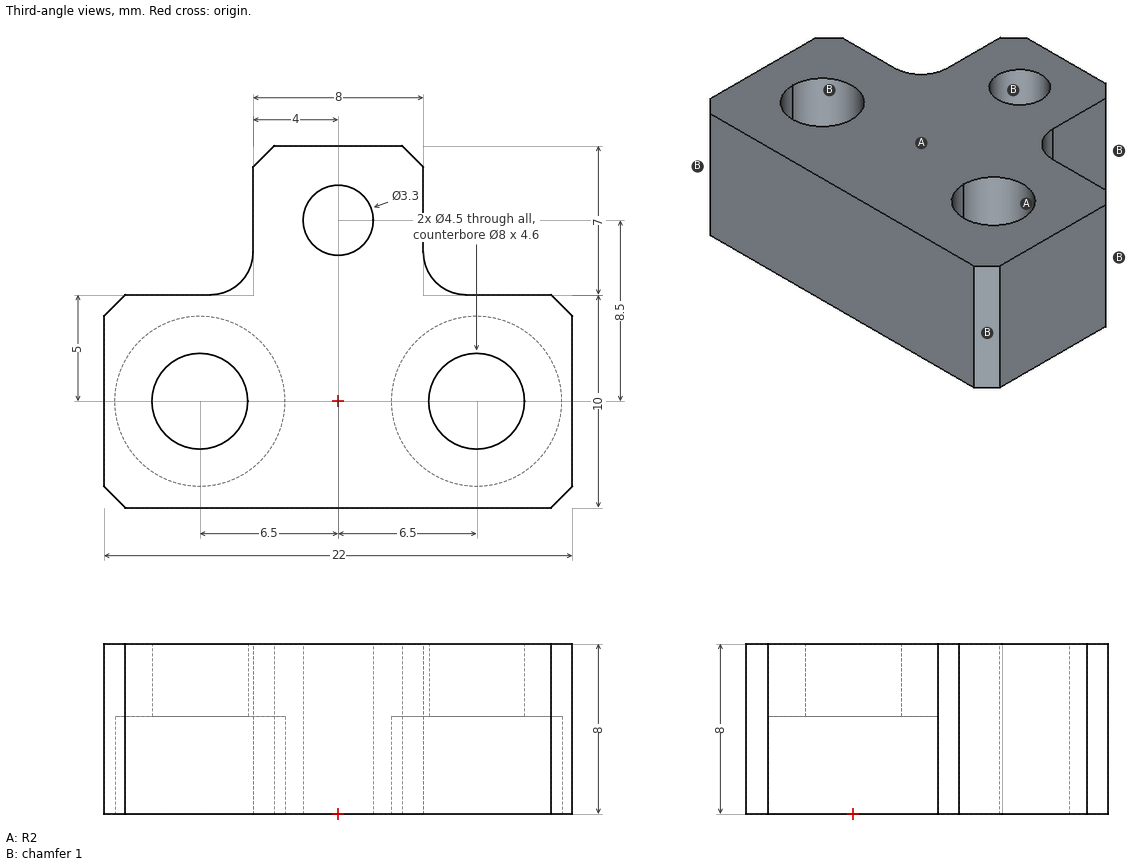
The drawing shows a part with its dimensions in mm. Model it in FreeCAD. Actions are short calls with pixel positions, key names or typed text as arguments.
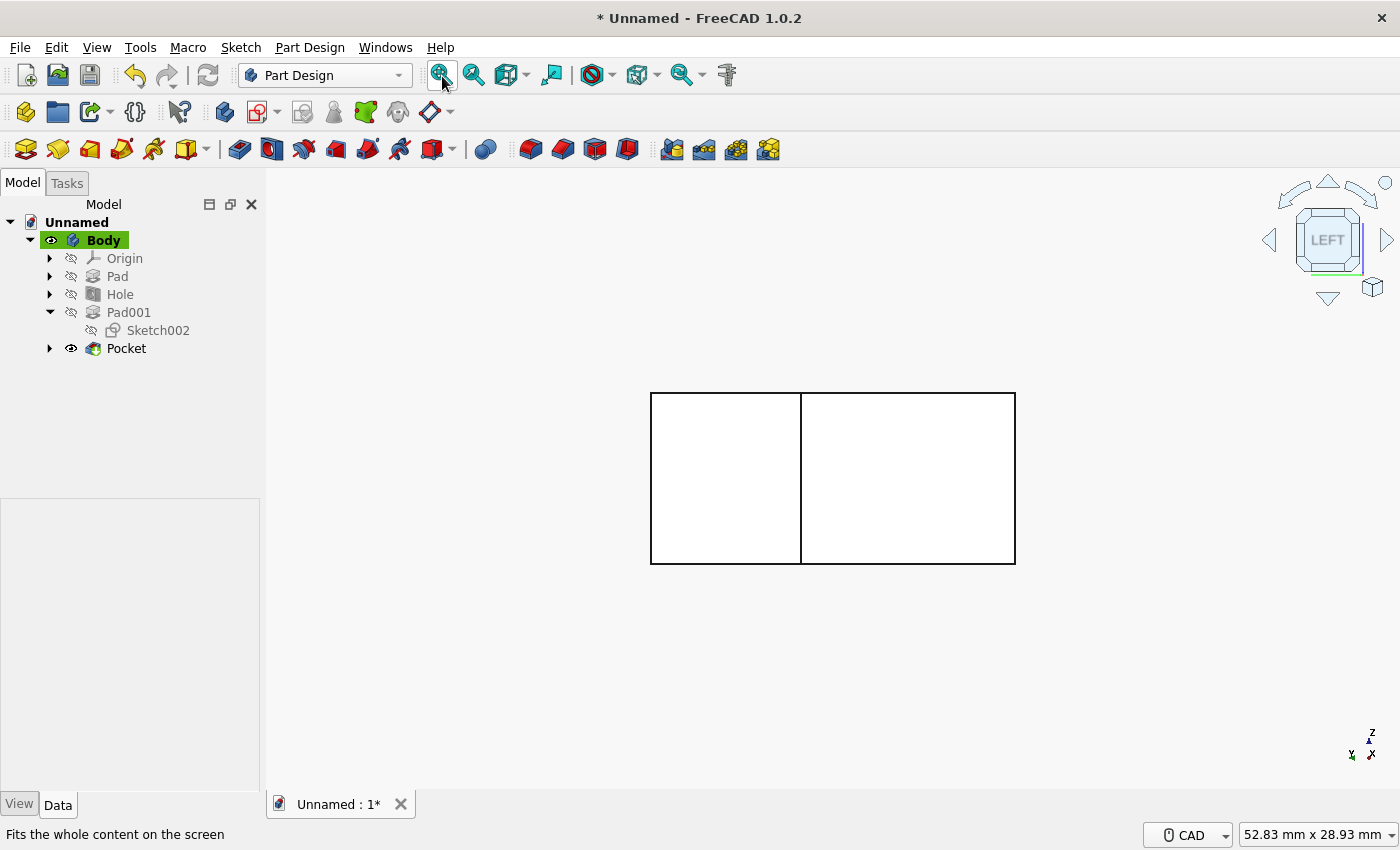
click(442, 76)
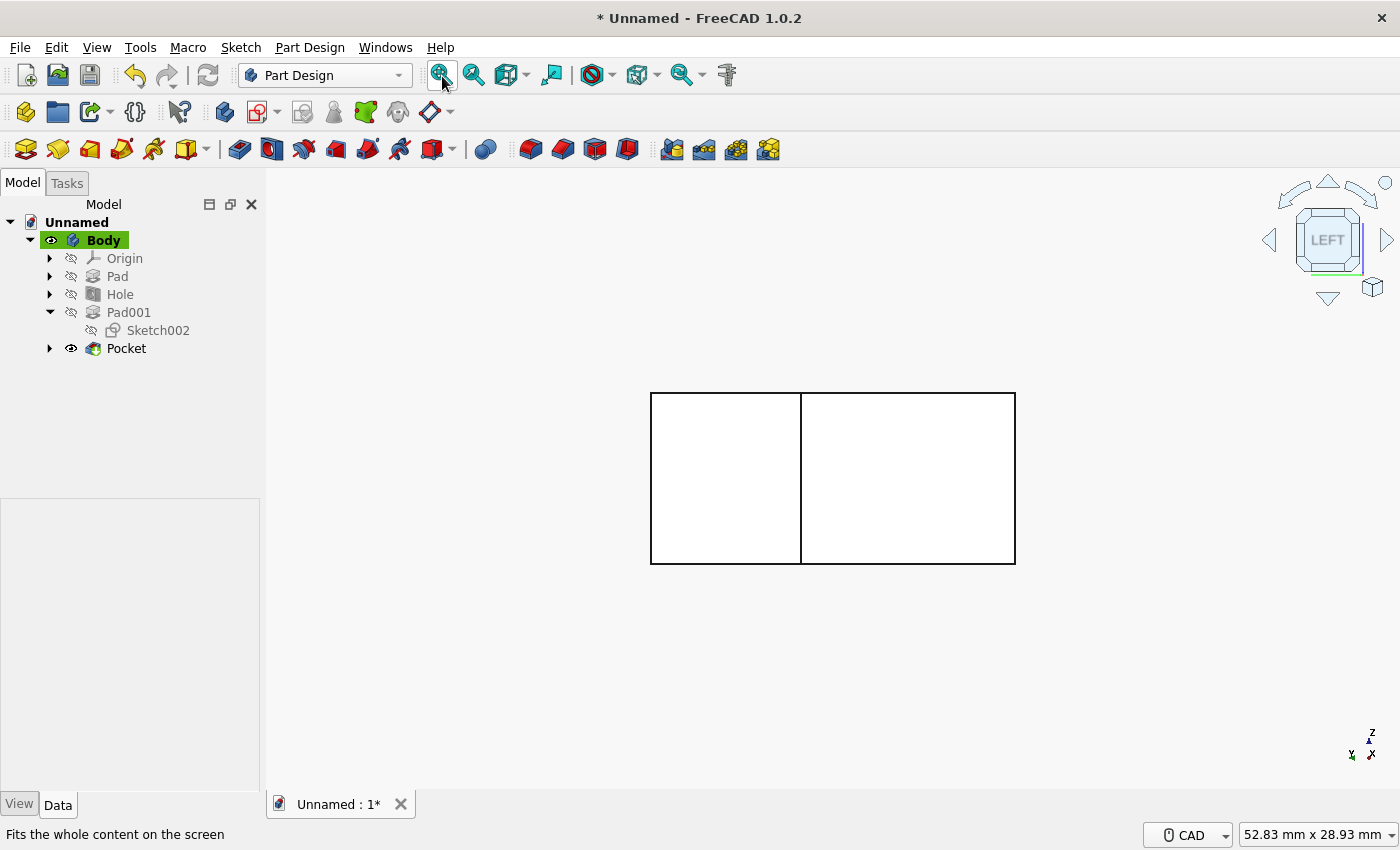
key(v)
key(3)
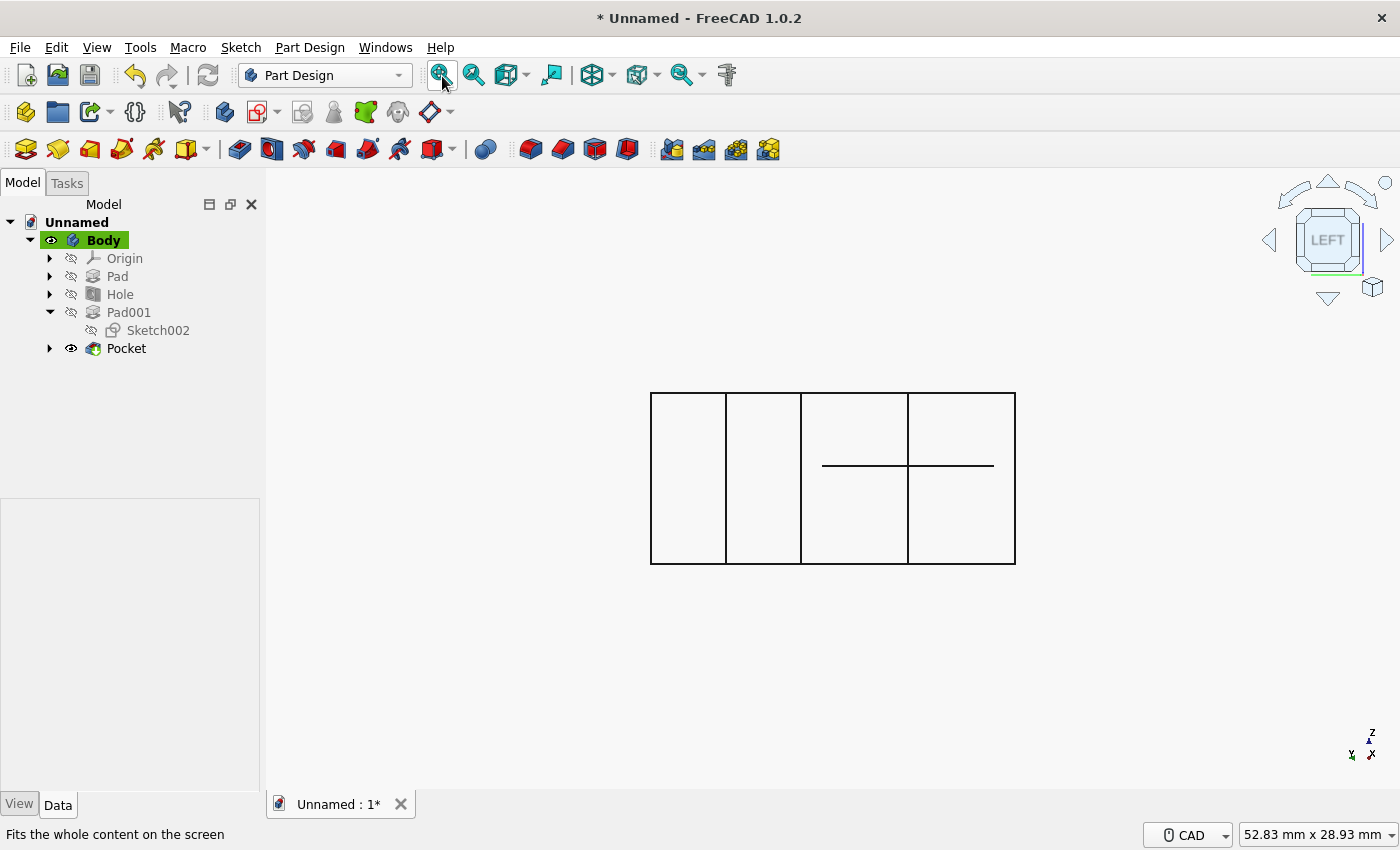
key(0)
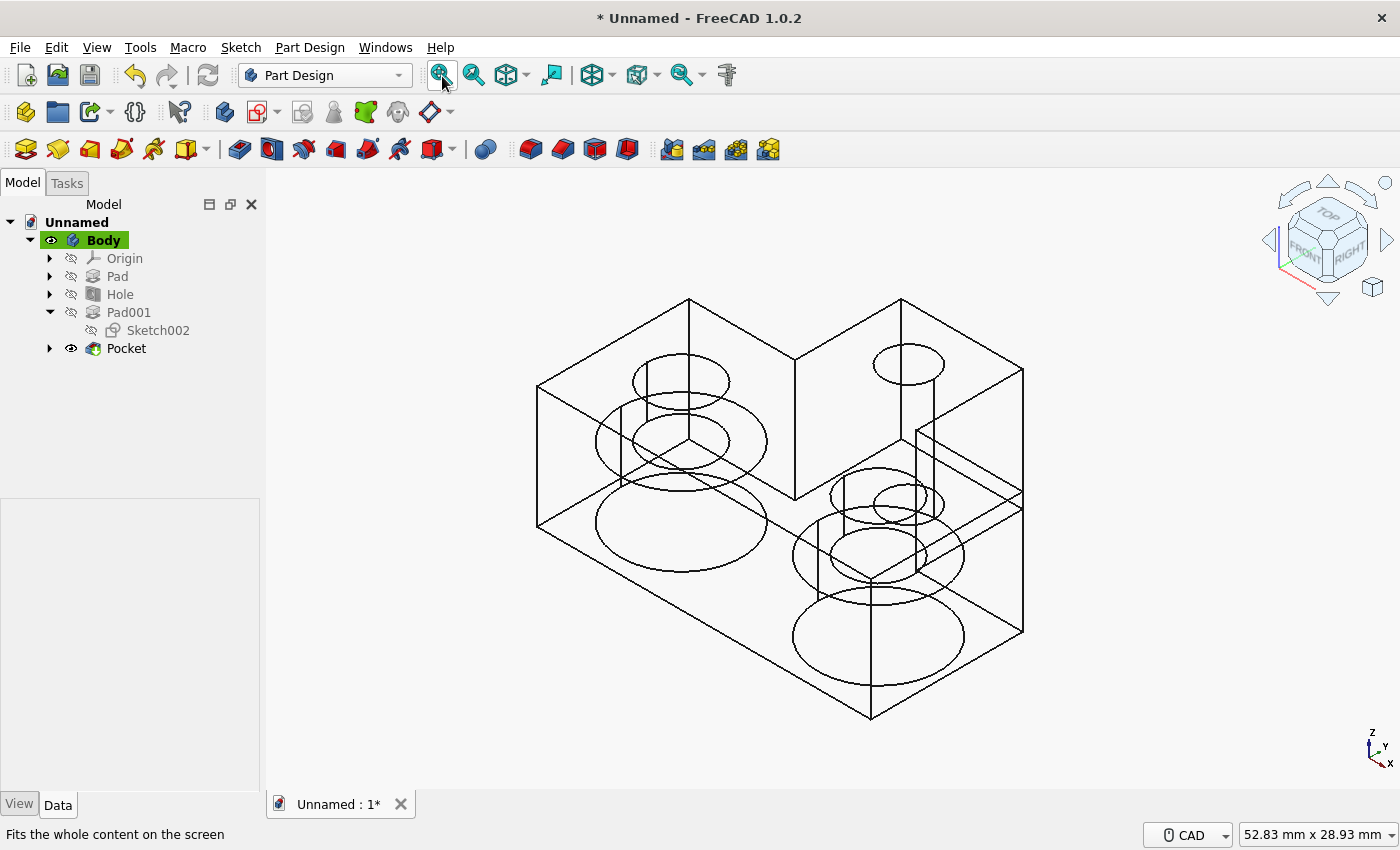
click(916, 499)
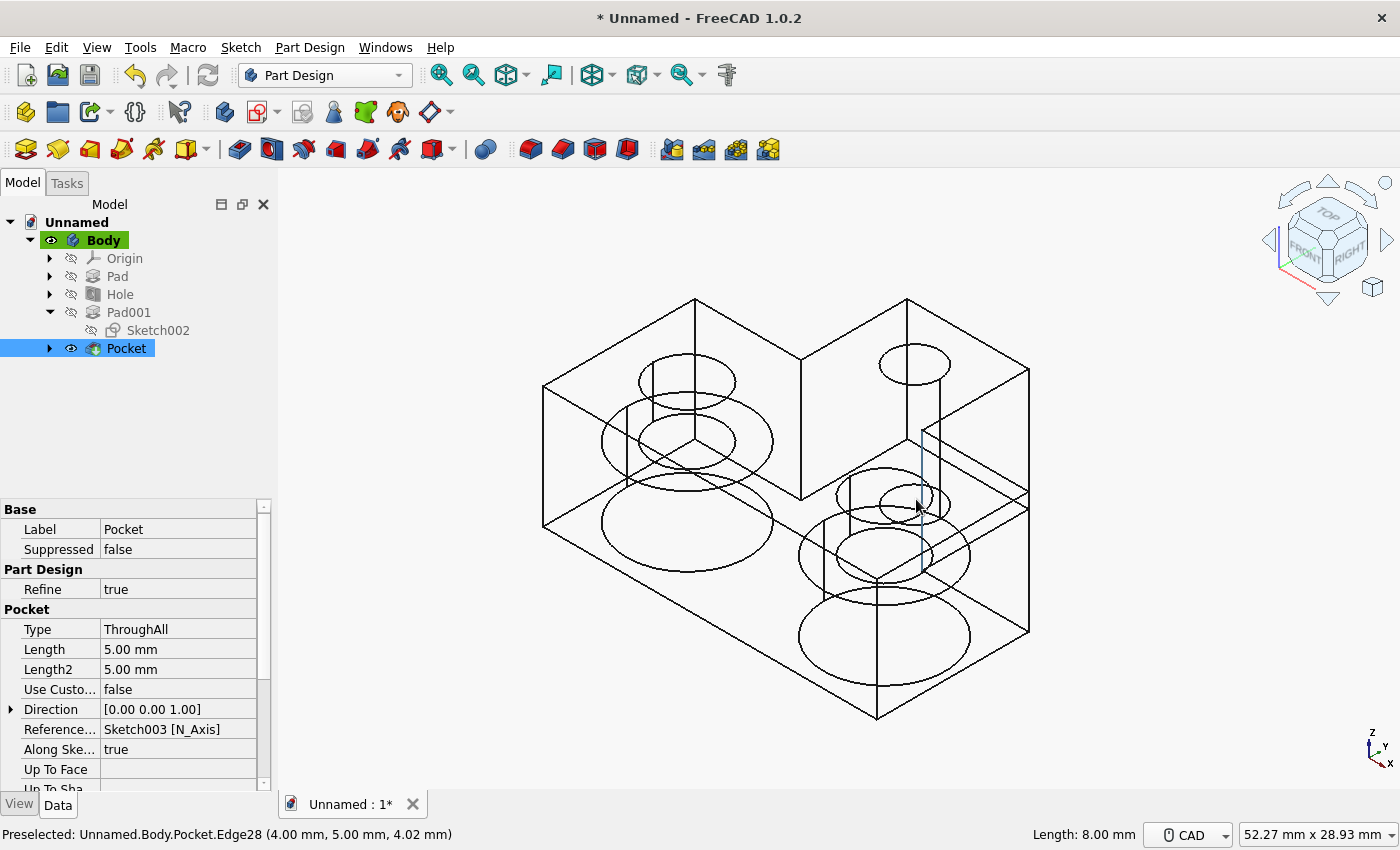
click(801, 429, ctrl)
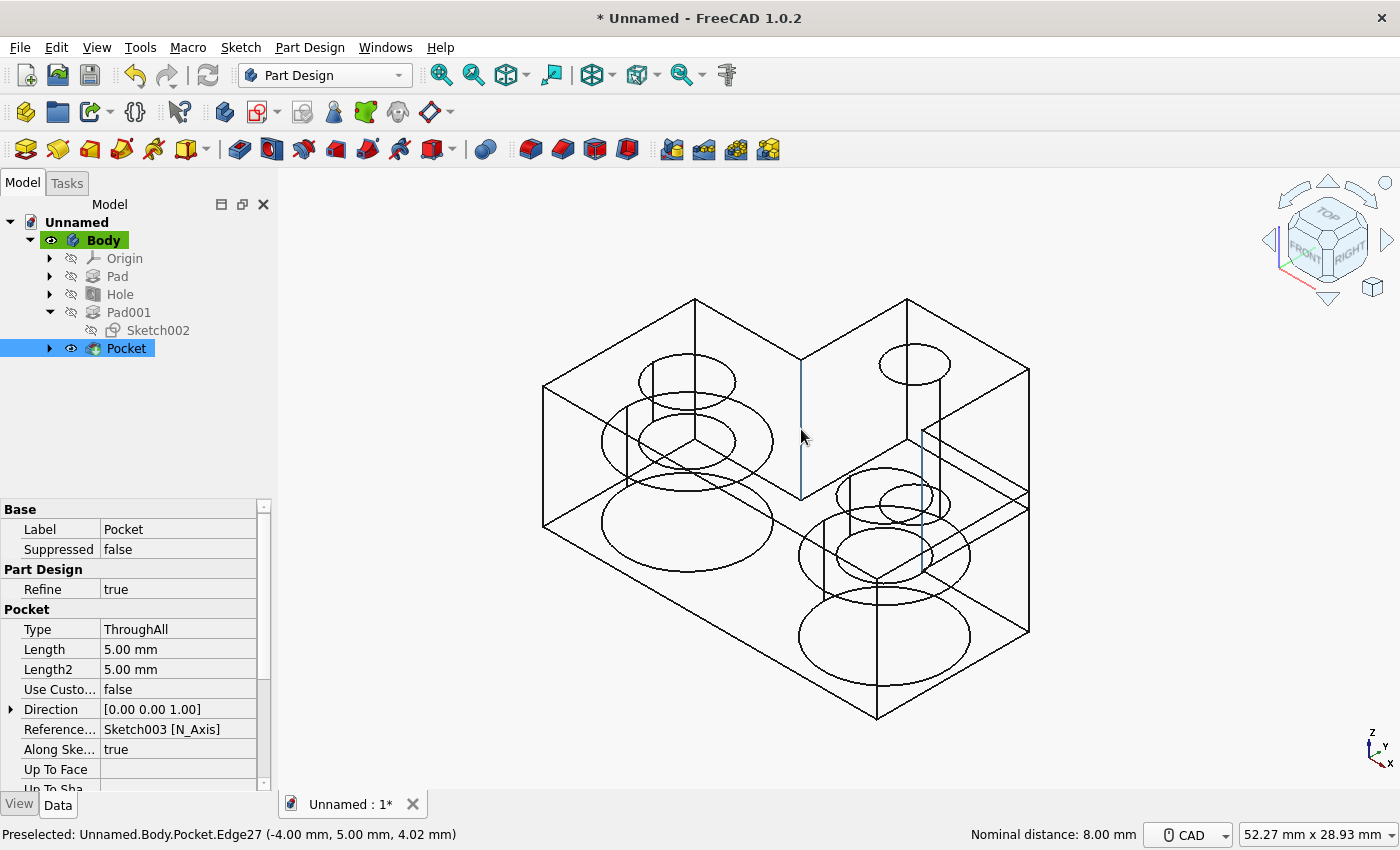
key(v)
key(1)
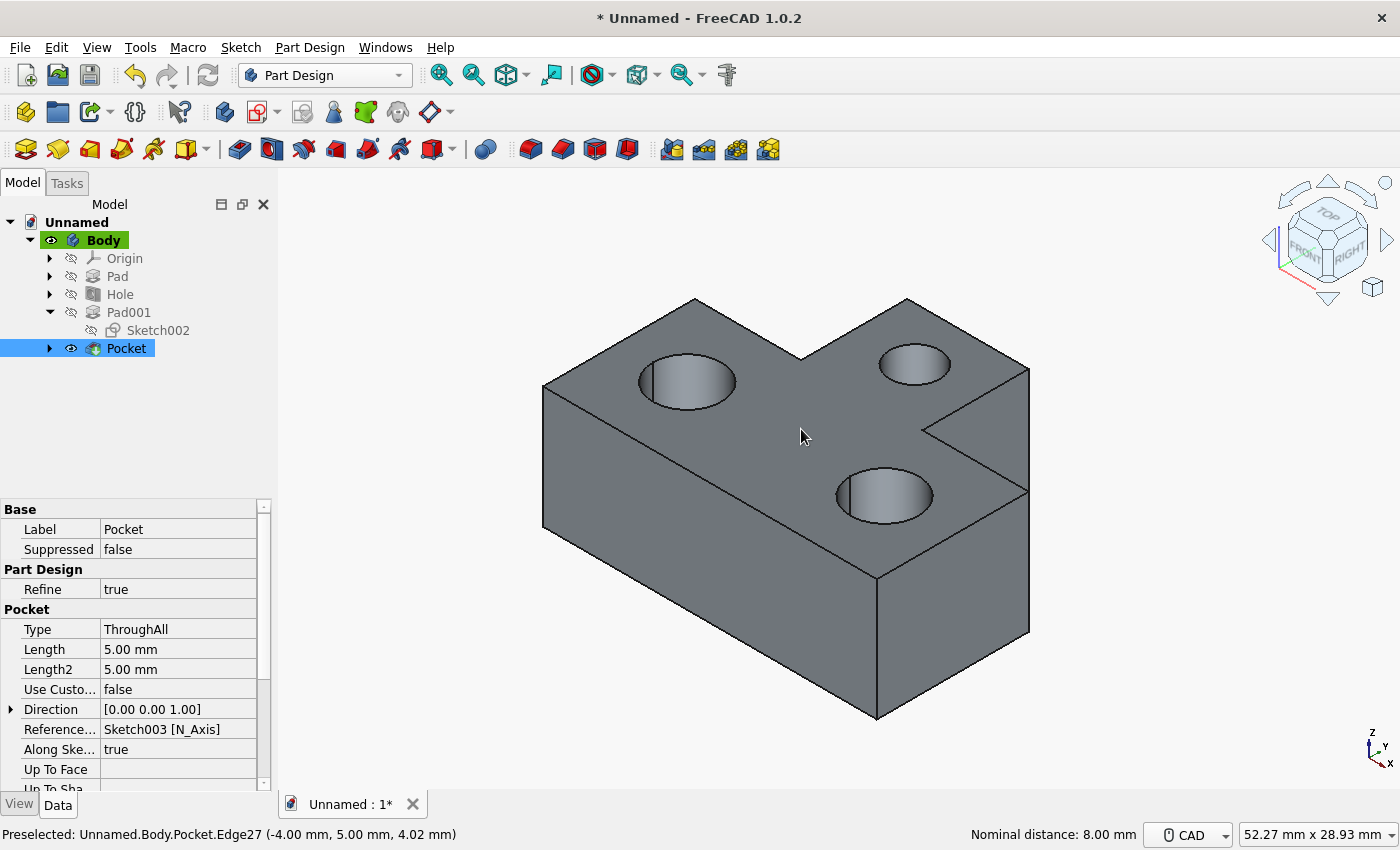
click(532, 150)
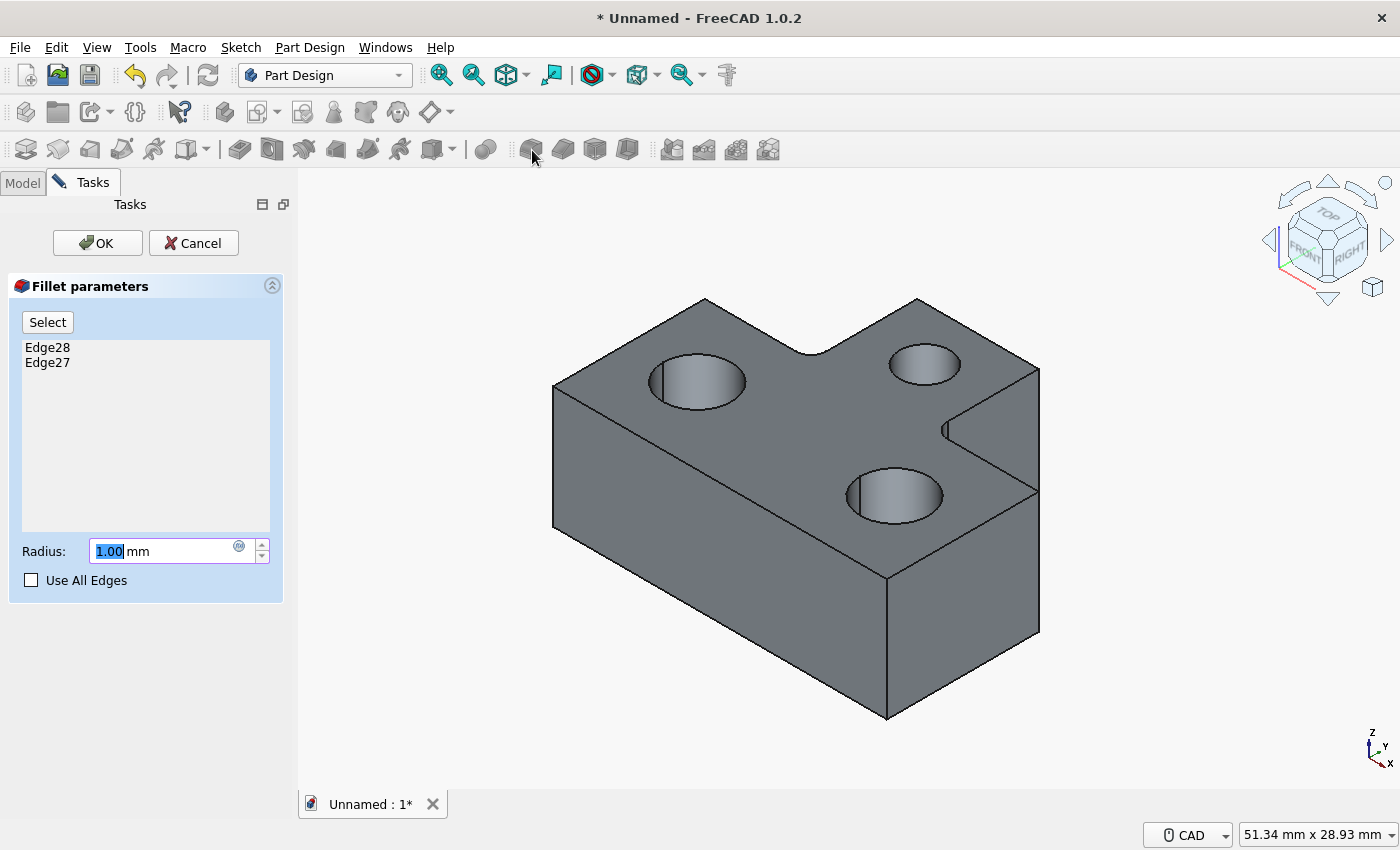
text(2)
key(Tab)